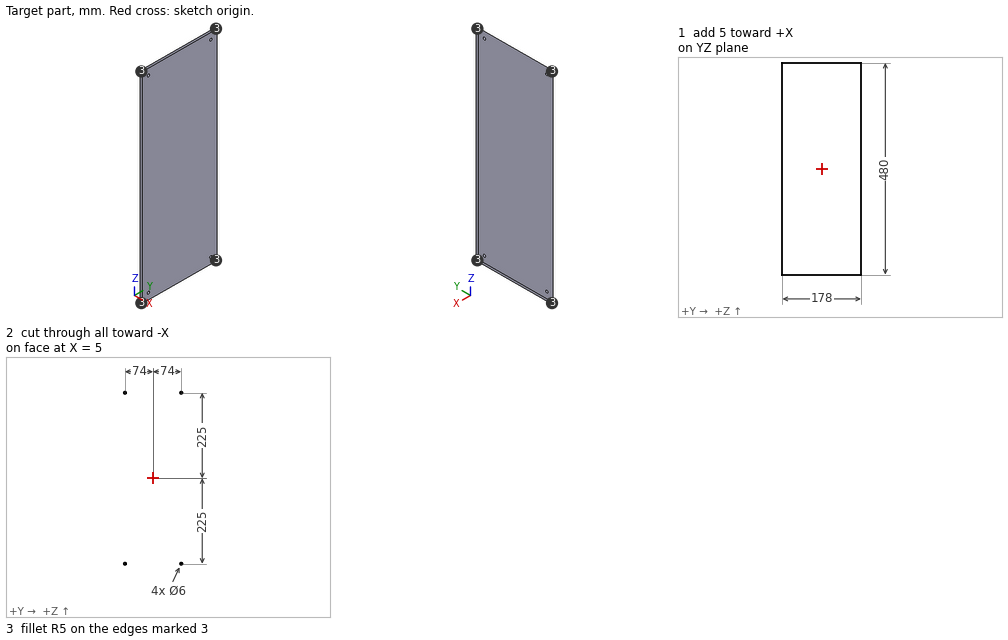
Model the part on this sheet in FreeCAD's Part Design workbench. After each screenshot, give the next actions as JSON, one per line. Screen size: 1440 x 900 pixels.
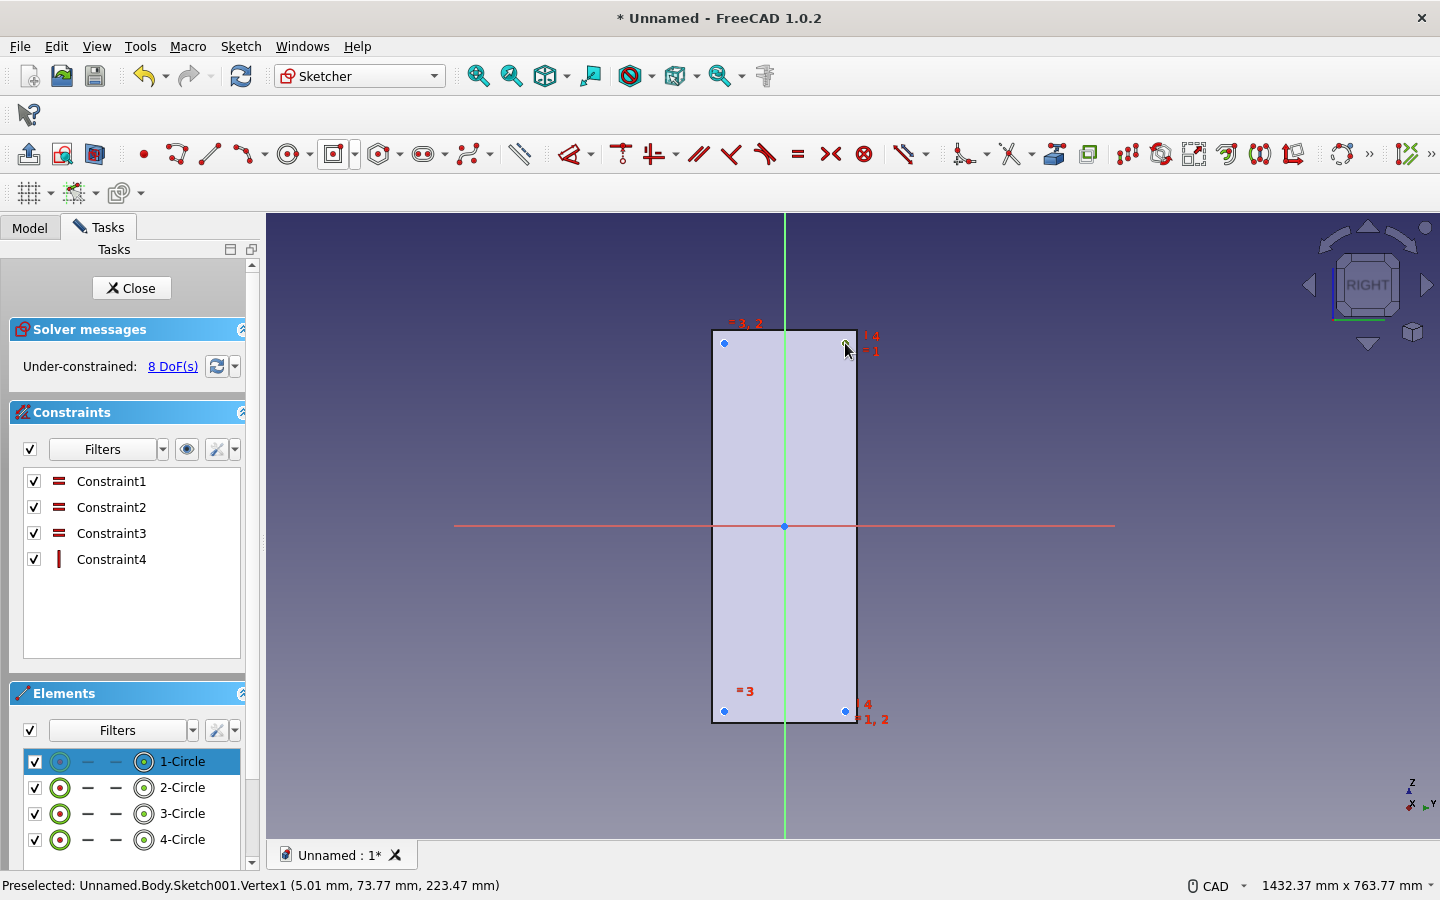
{"action": "left_click", "coordinate": [724, 343]}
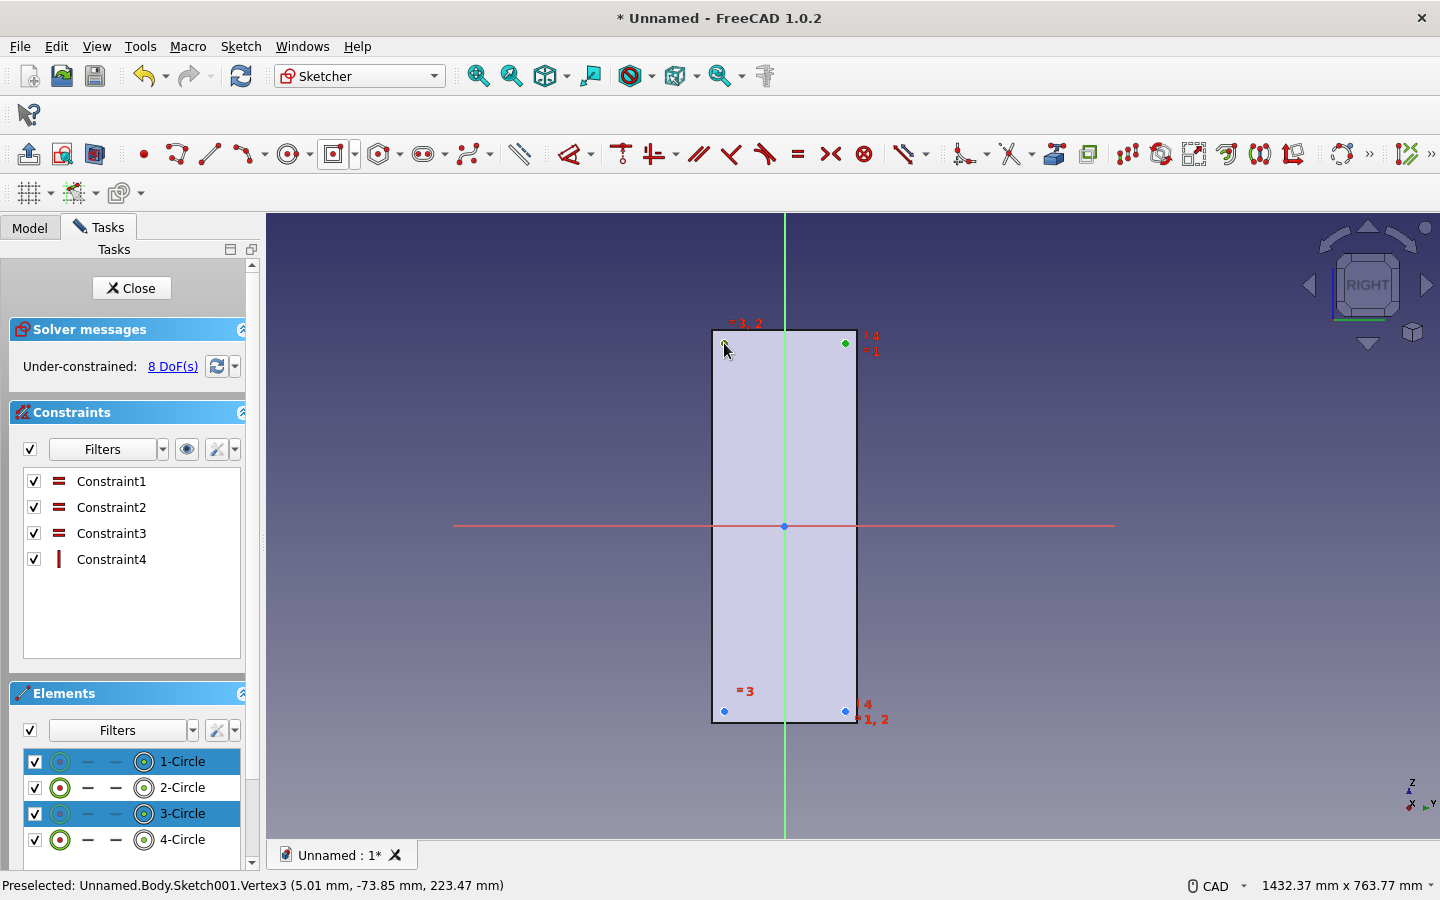
{"action": "left_click", "coordinate": [676, 154]}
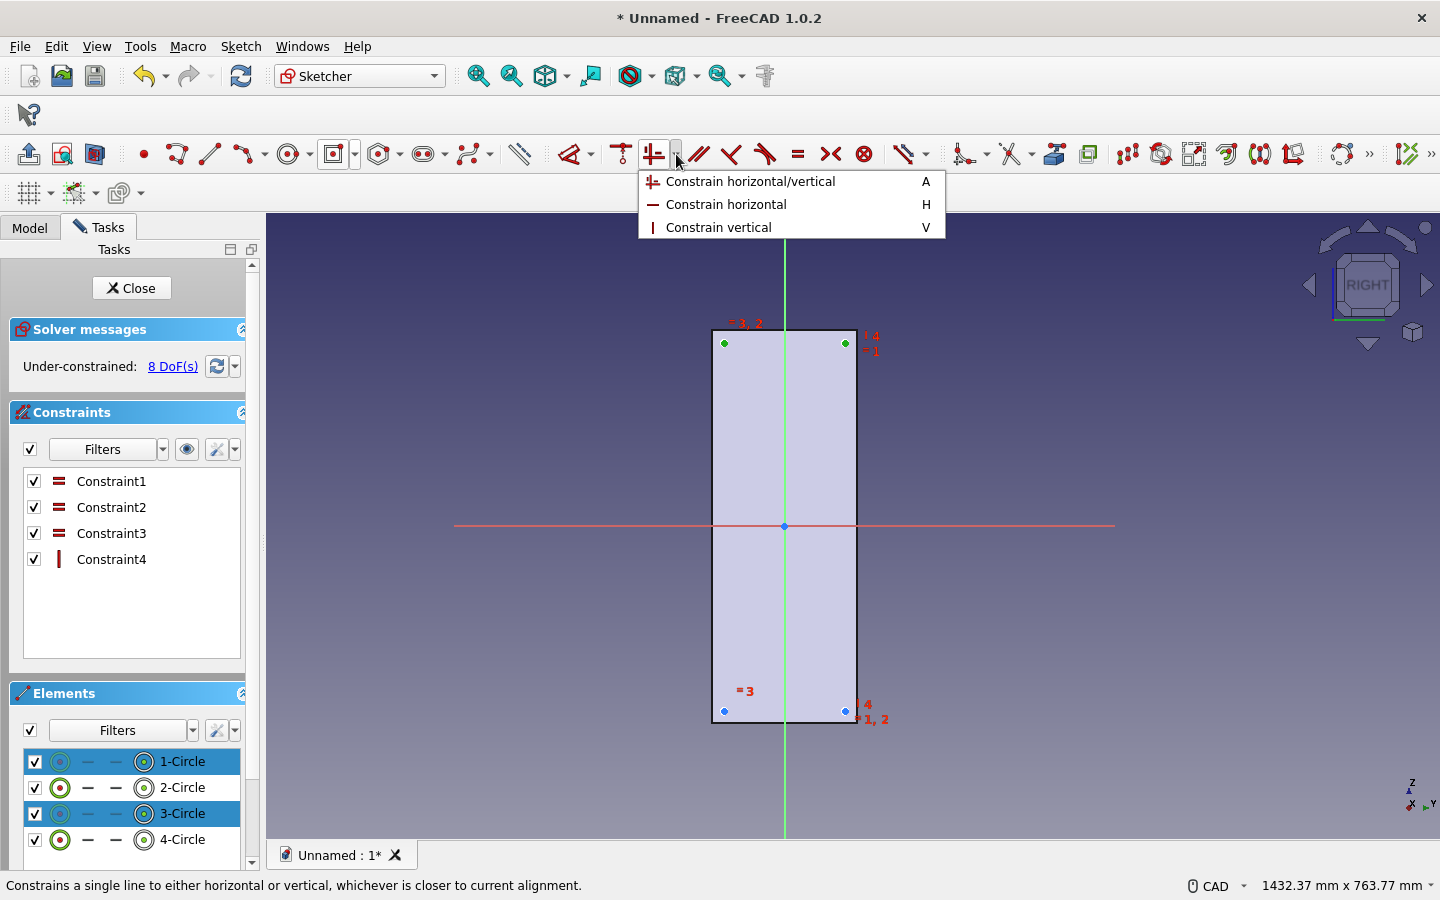
{"action": "left_click", "coordinate": [792, 204]}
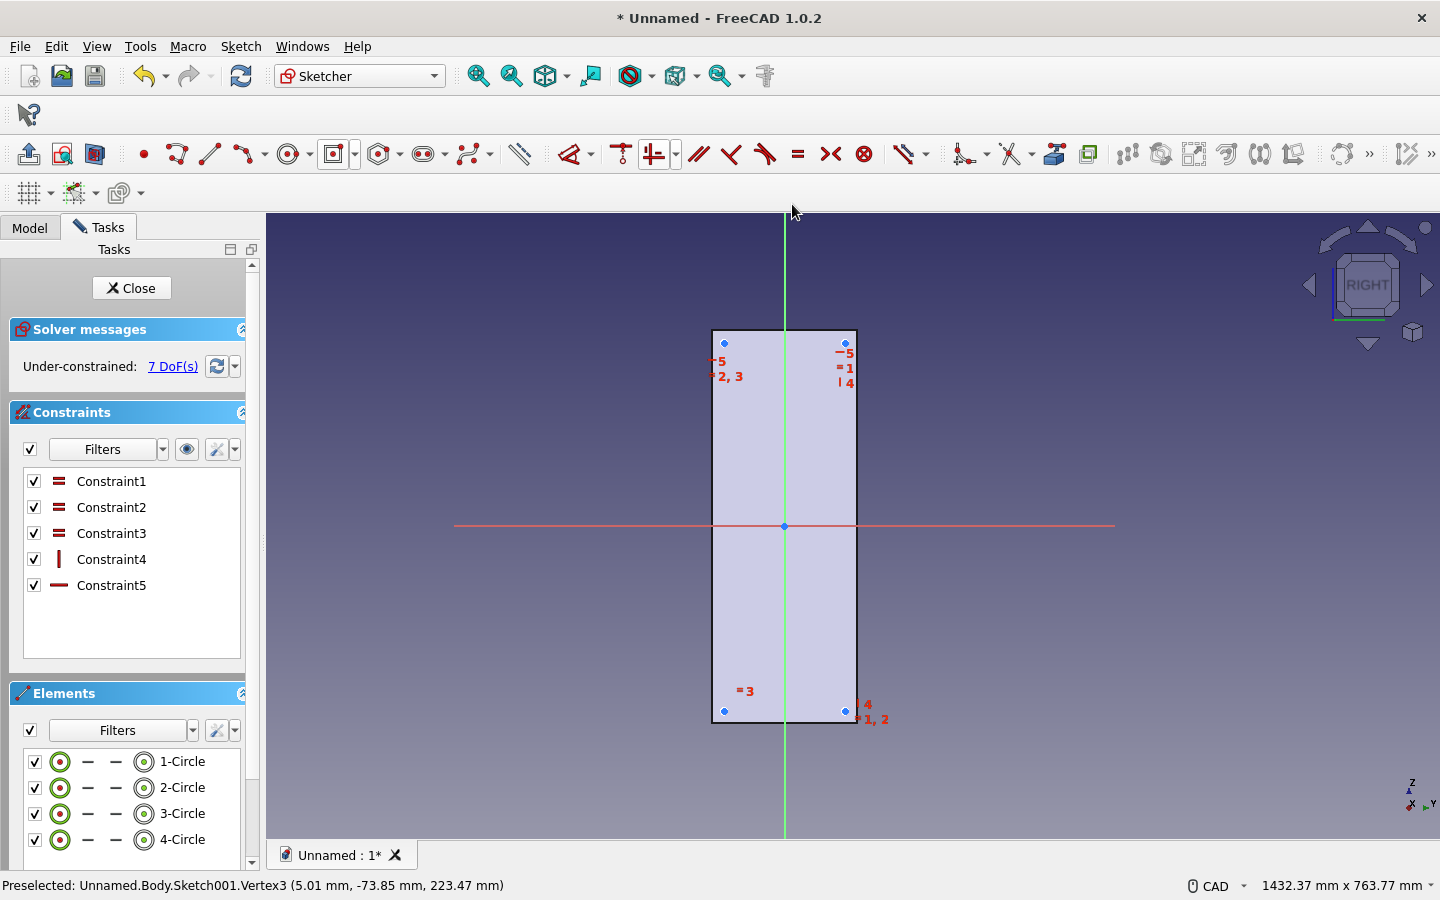
{"action": "left_click", "coordinate": [724, 343]}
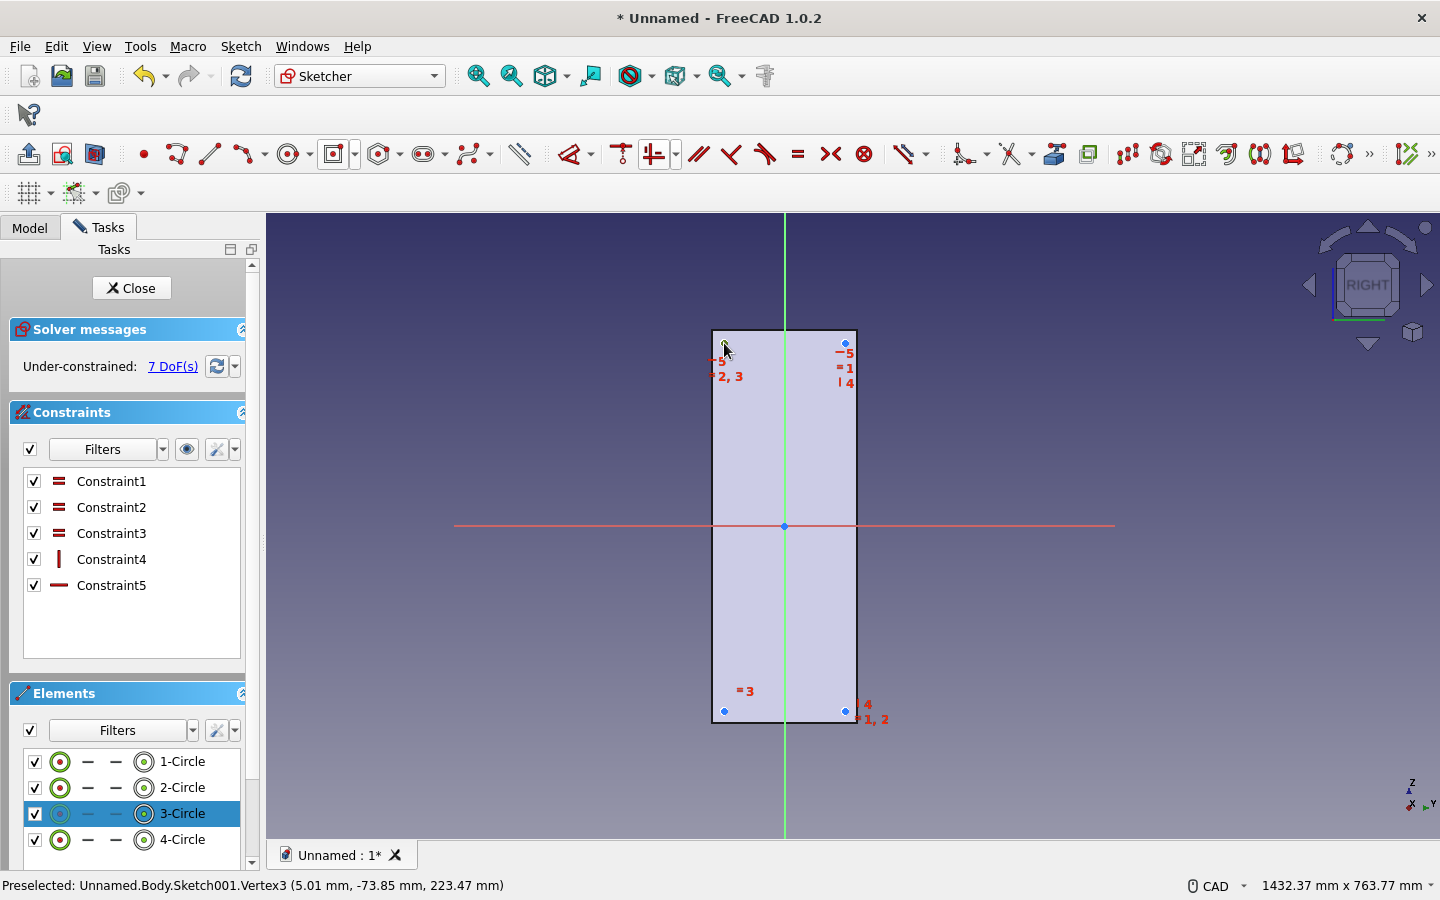
{"action": "left_click", "coordinate": [724, 711]}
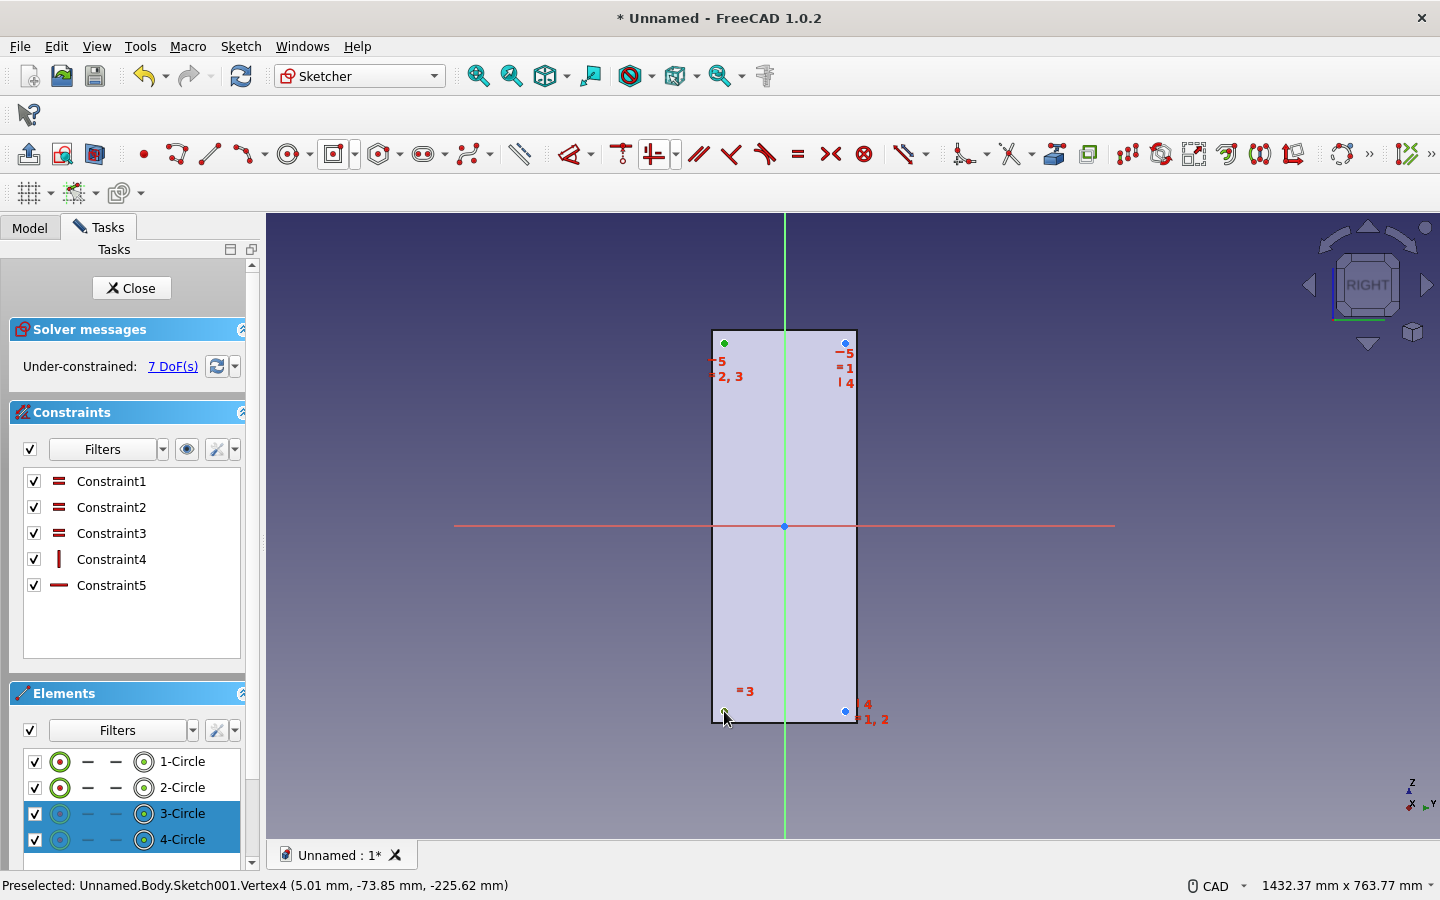
{"action": "left_click", "coordinate": [676, 154]}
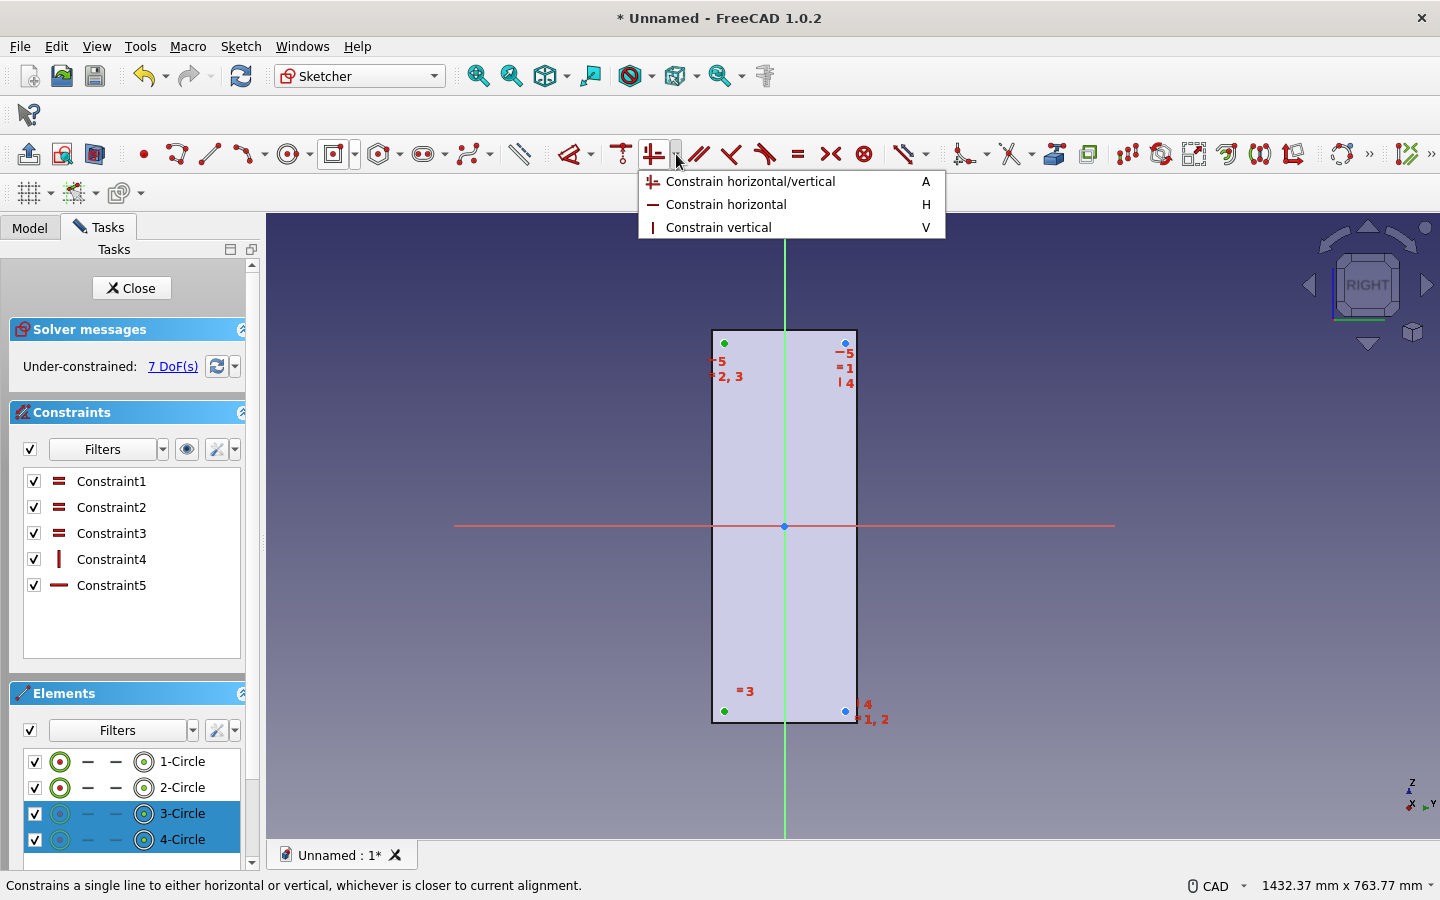
{"action": "left_click", "coordinate": [792, 228]}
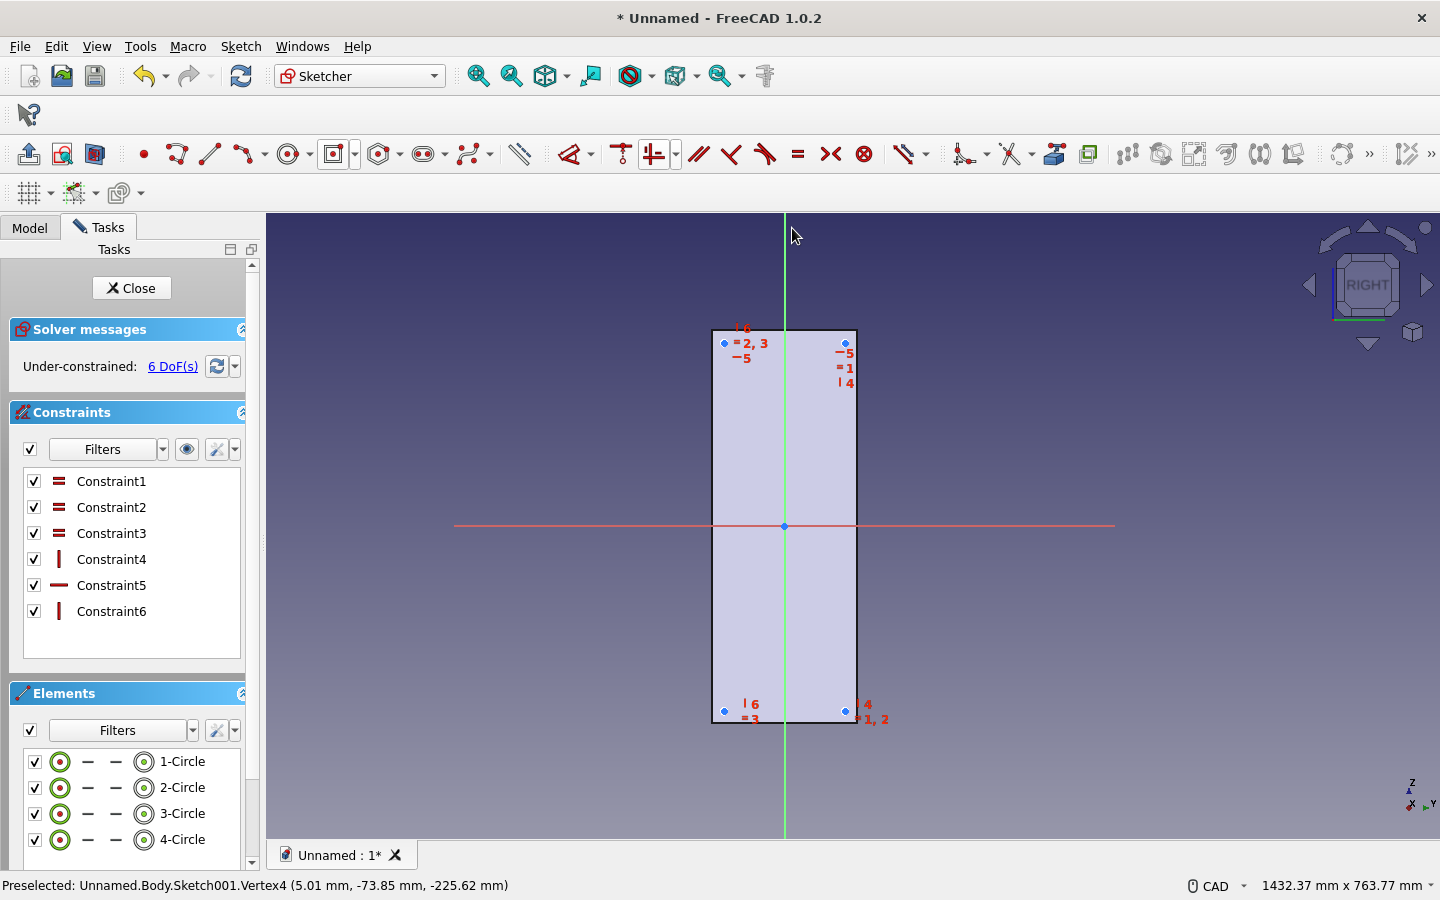
{"action": "left_click", "coordinate": [845, 711]}